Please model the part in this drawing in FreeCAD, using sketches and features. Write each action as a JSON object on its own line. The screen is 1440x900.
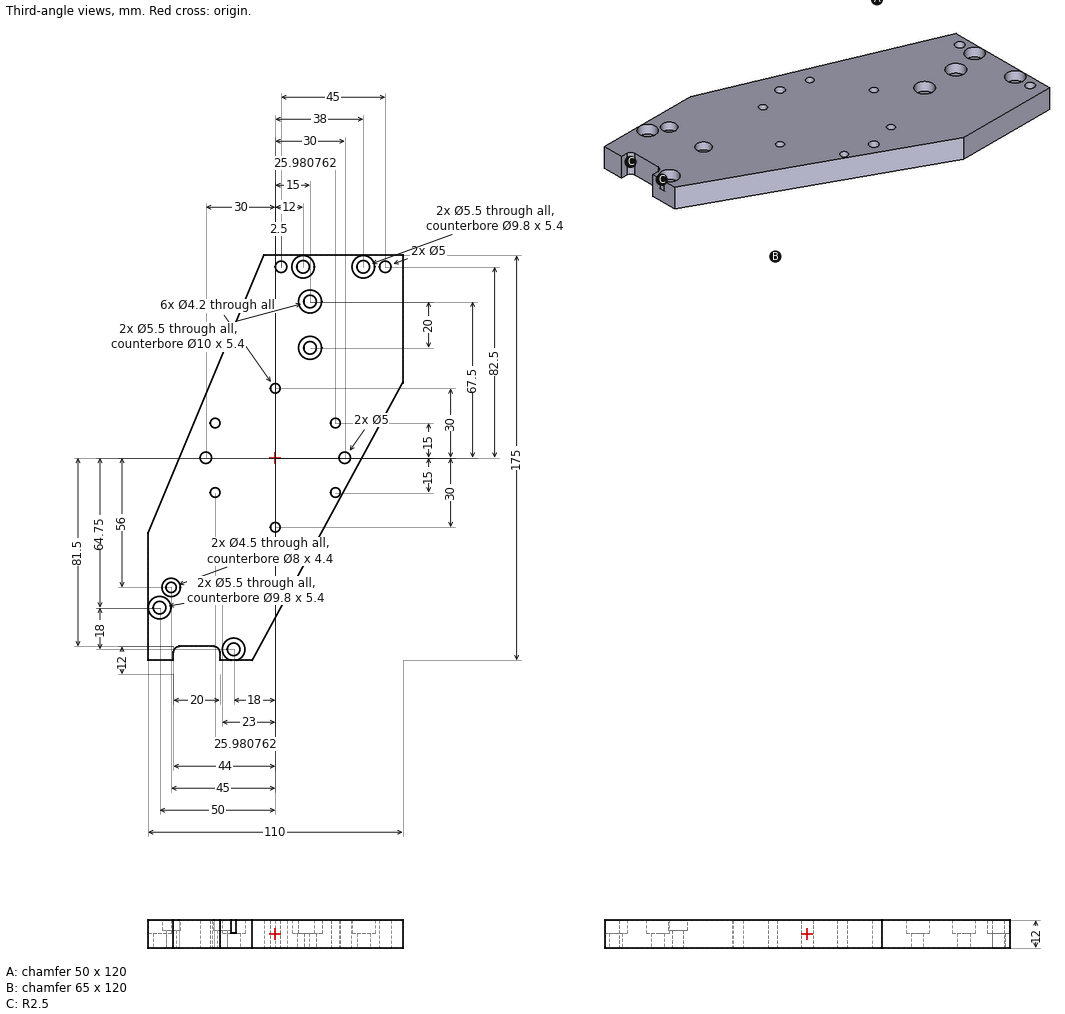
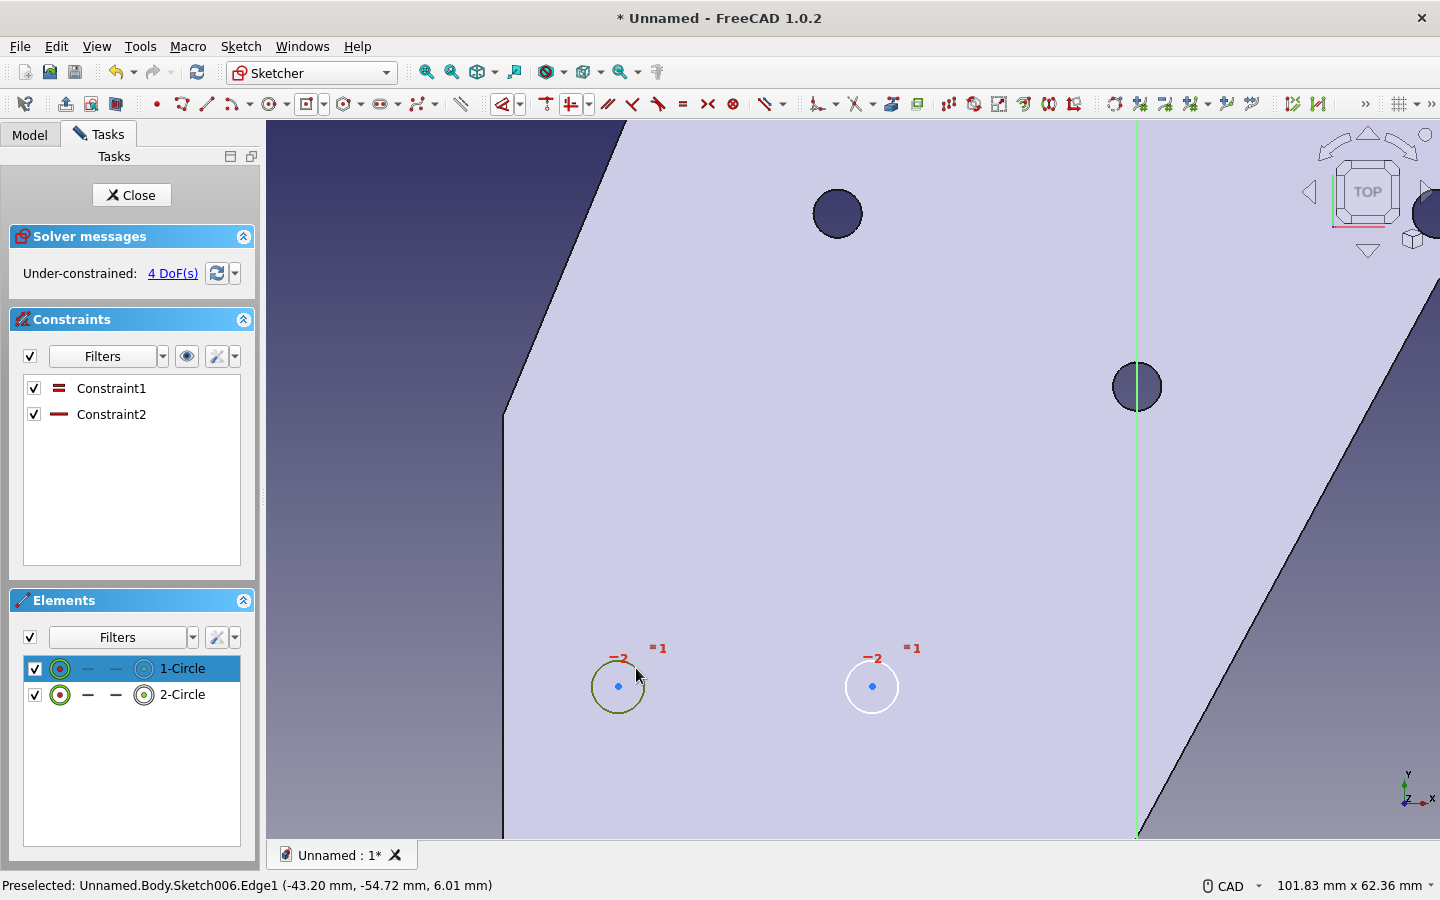
{"action": "key", "text": "k o"}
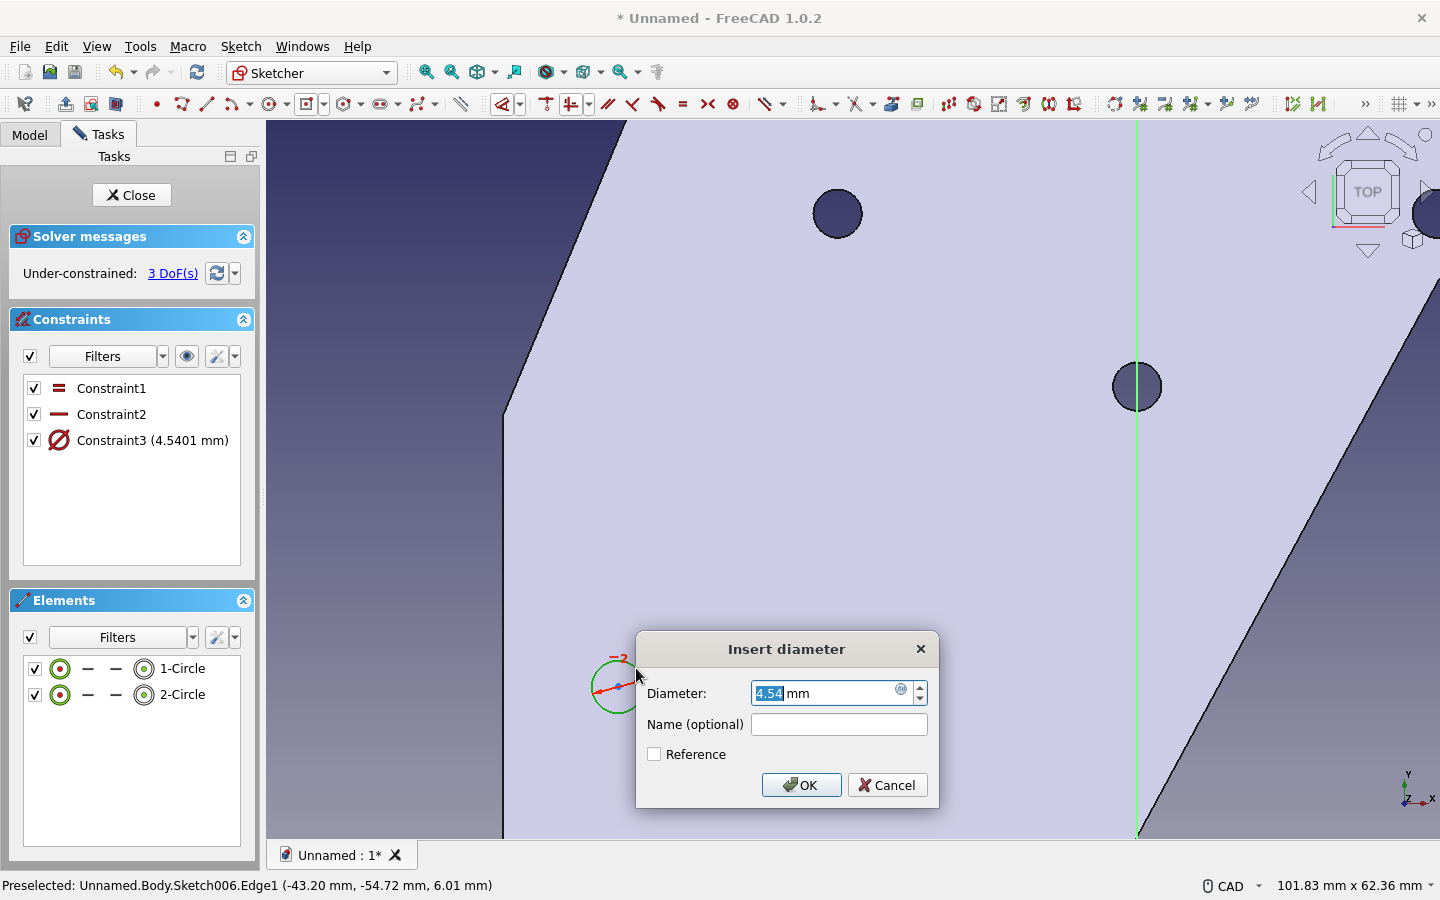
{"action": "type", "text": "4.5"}
{"action": "key", "text": "Return"}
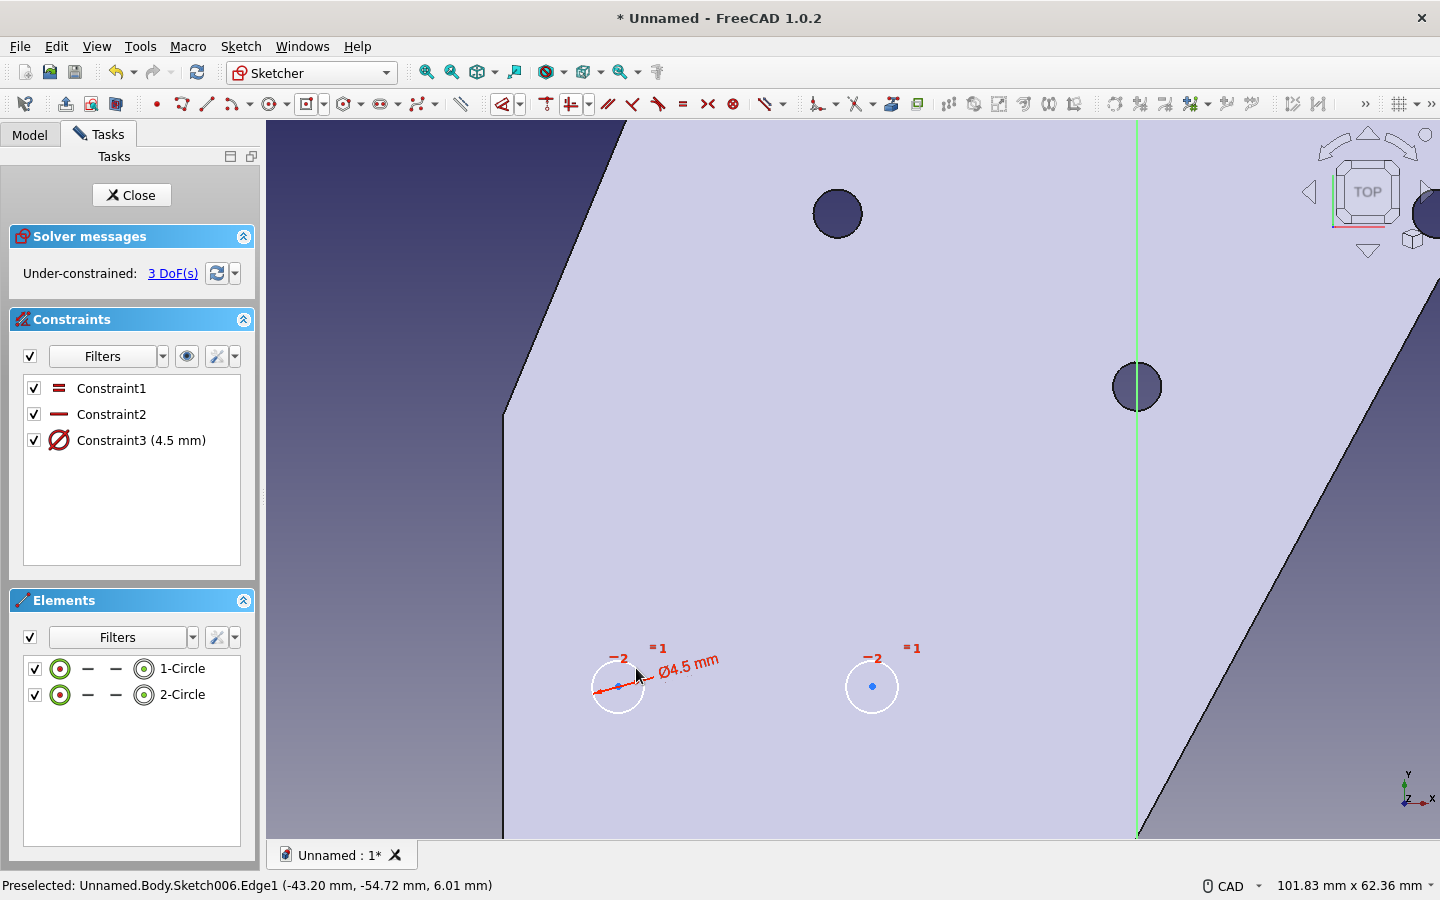
{"action": "left_click", "coordinate": [618, 687]}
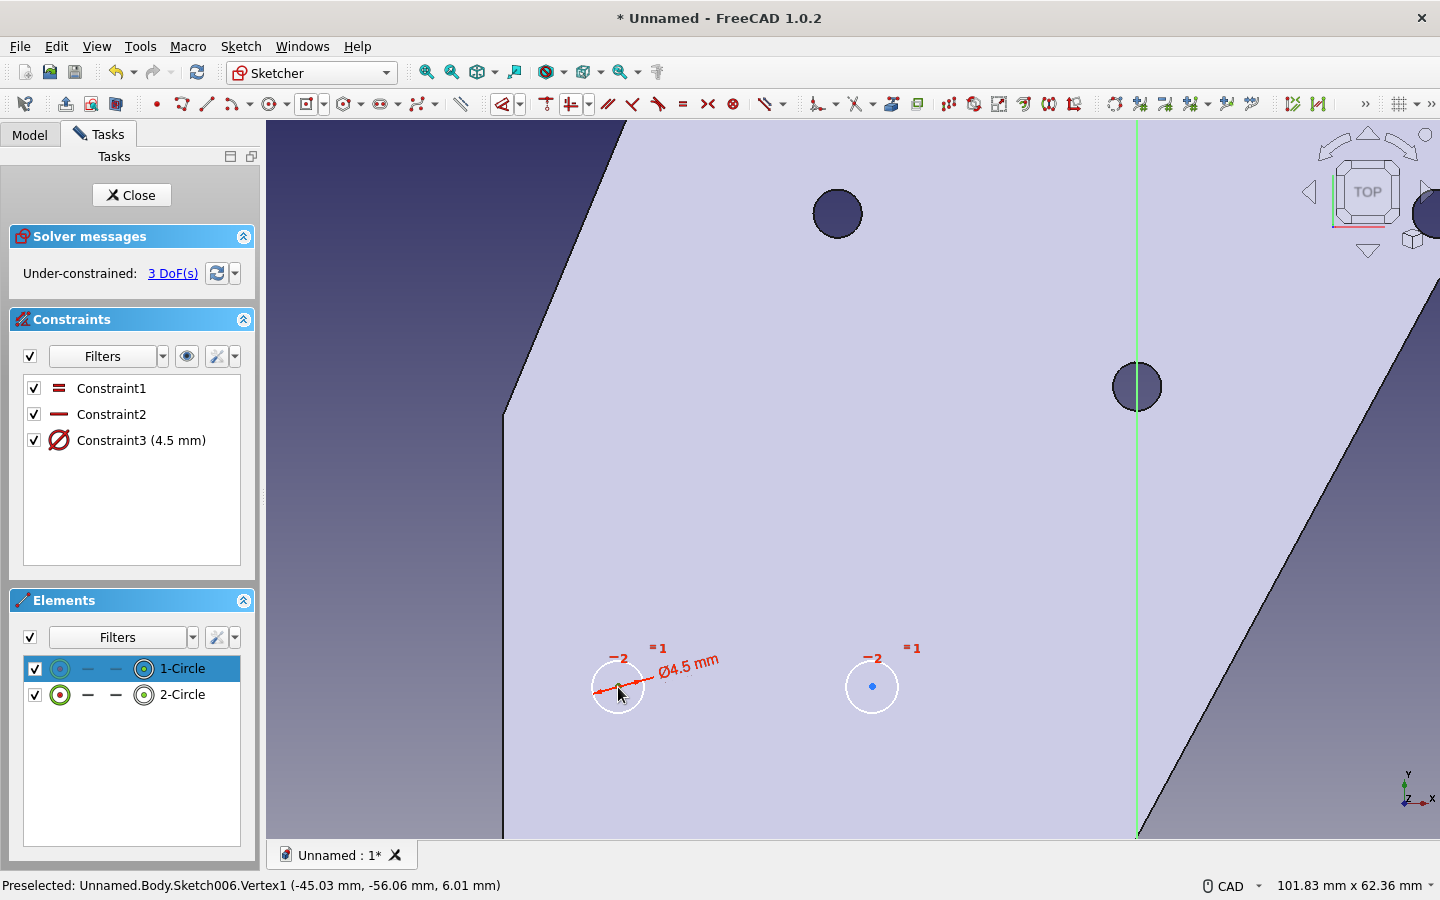
{"action": "key", "text": "l"}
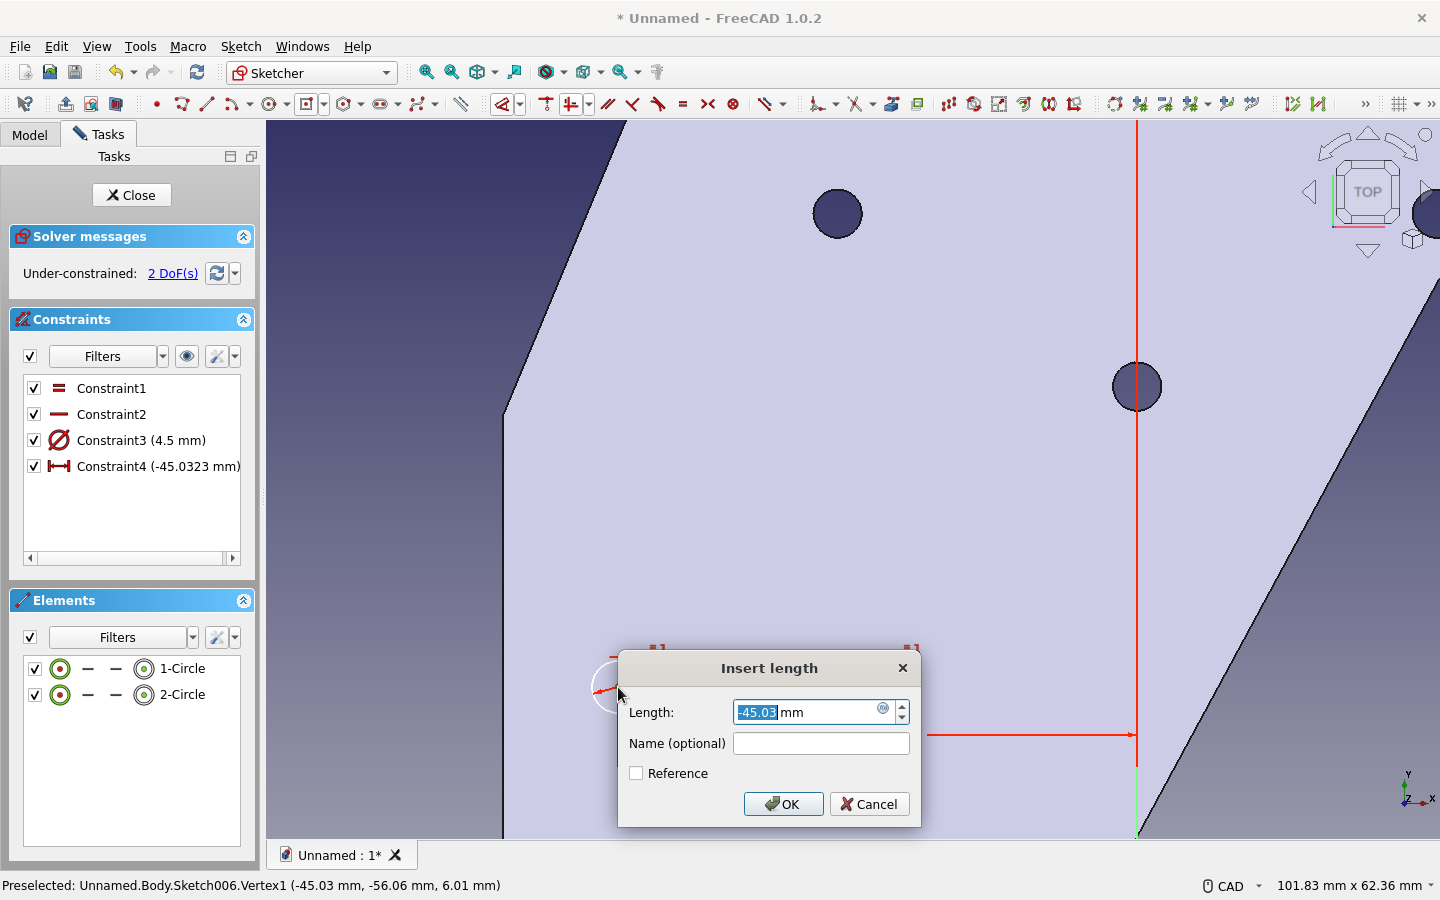
{"action": "type", "text": "-45"}
{"action": "key", "text": "Return"}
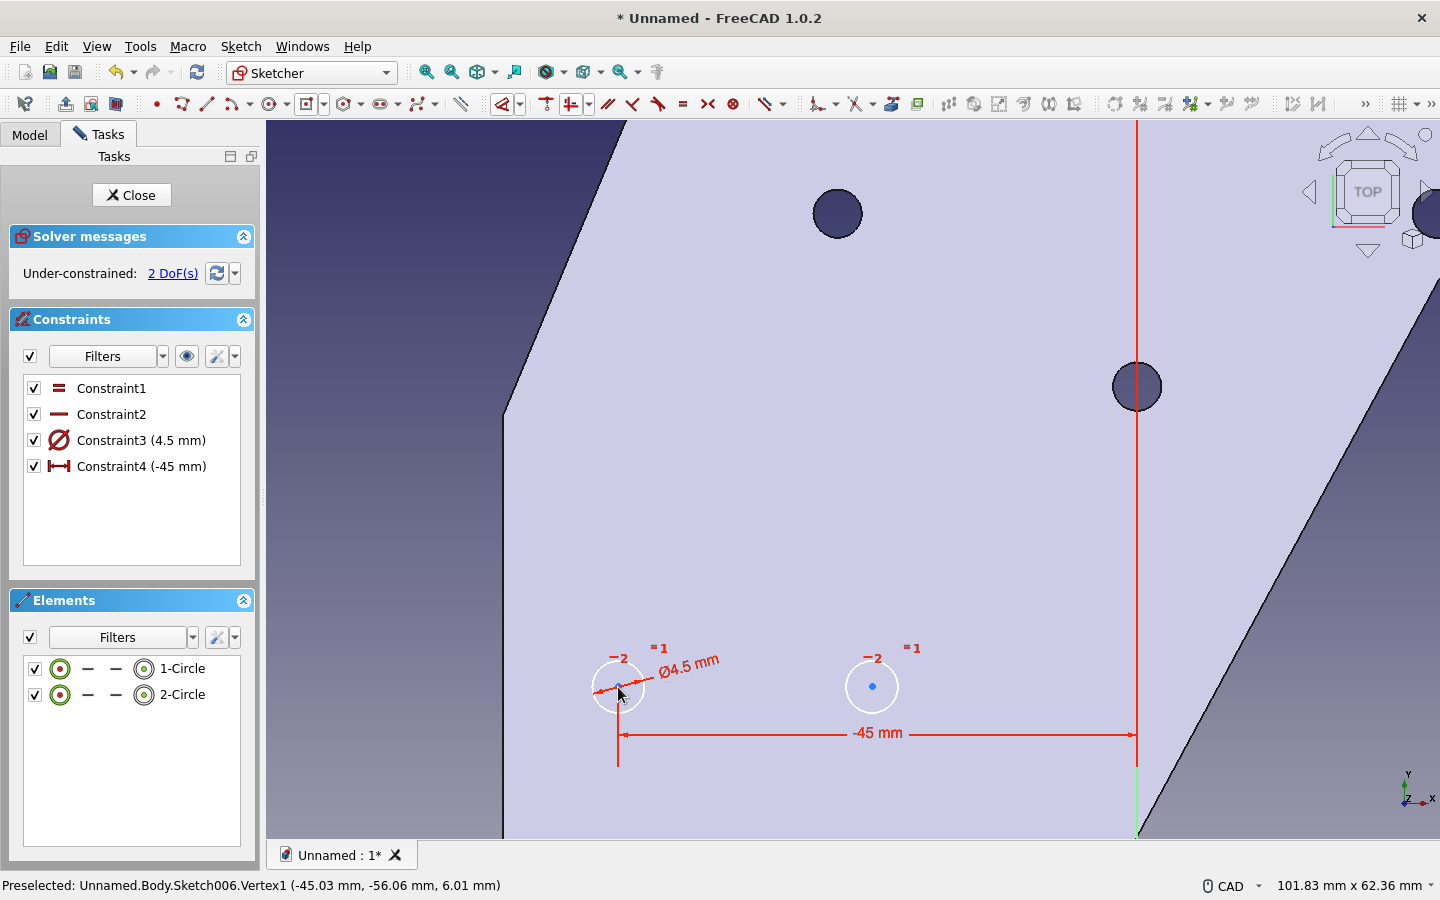
{"action": "left_click", "coordinate": [618, 687]}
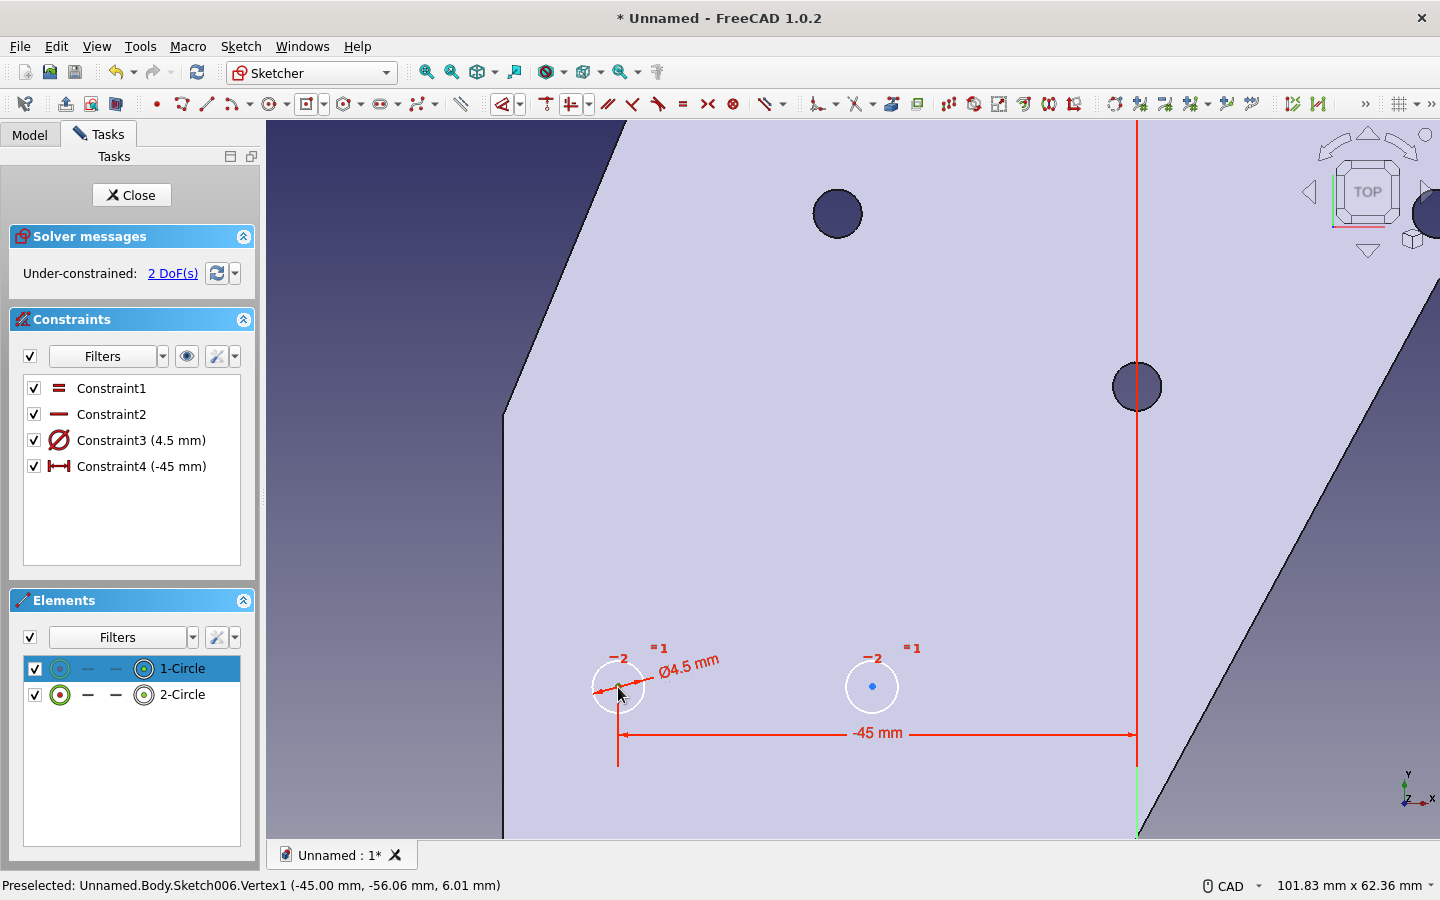
{"action": "key", "text": "i"}